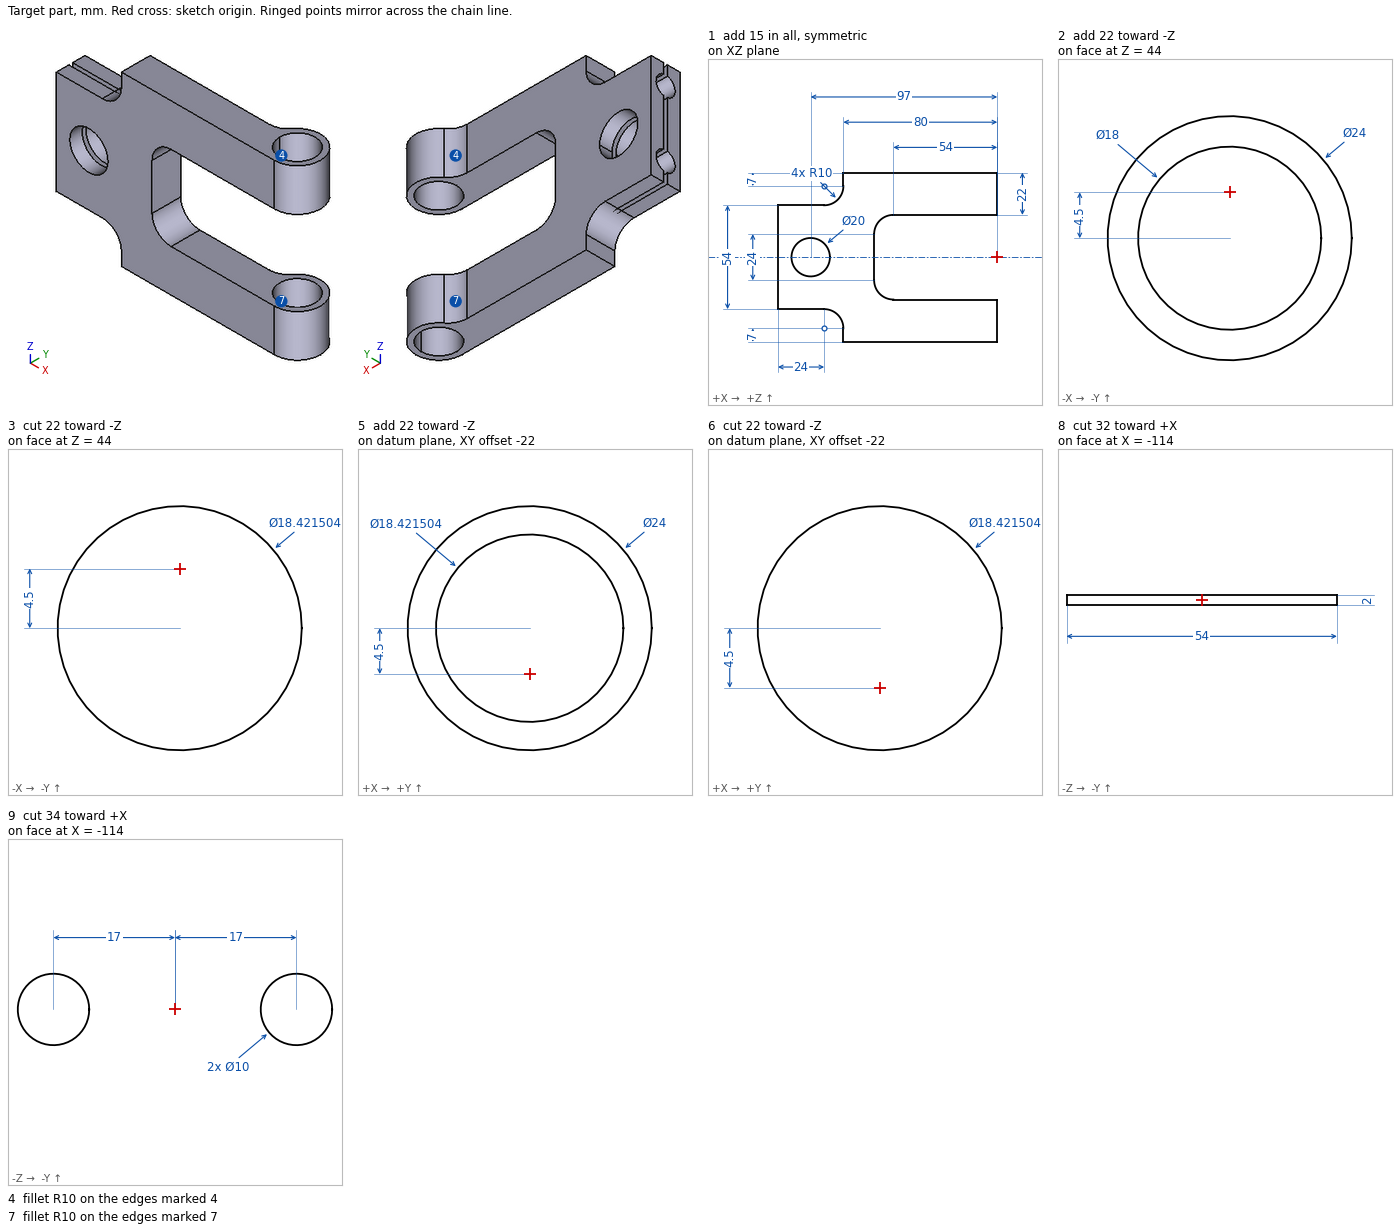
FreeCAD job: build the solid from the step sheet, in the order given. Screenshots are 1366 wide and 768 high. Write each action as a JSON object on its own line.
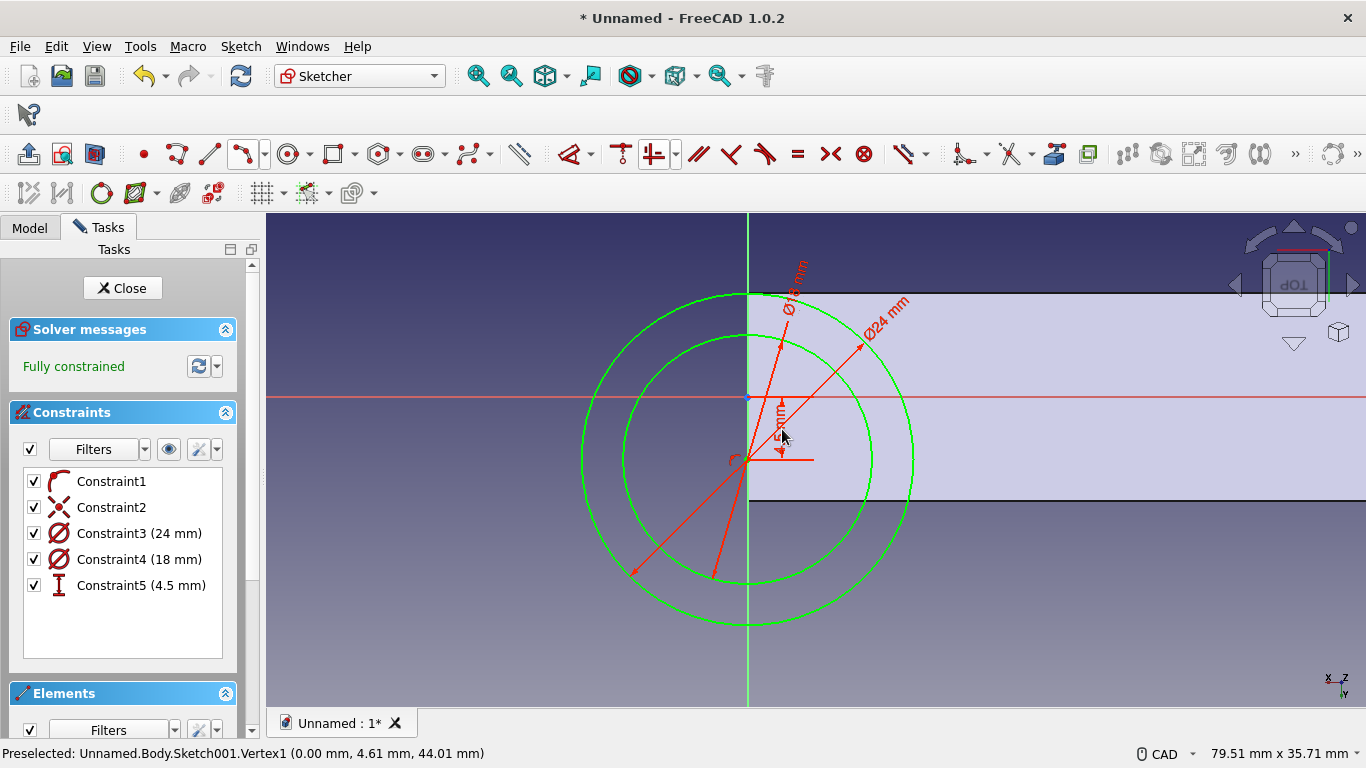
{"action": "left_click", "coordinate": [123, 288]}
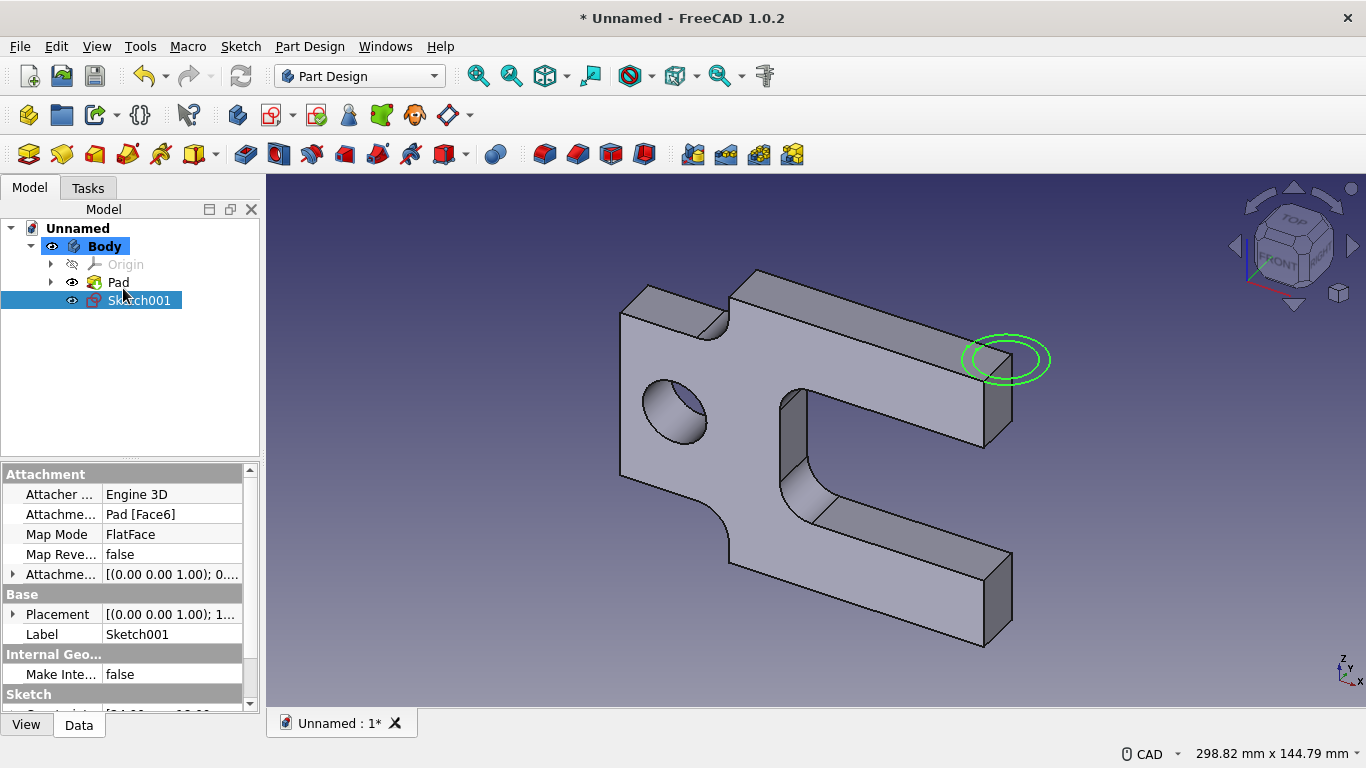
{"action": "left_click", "coordinate": [29, 154]}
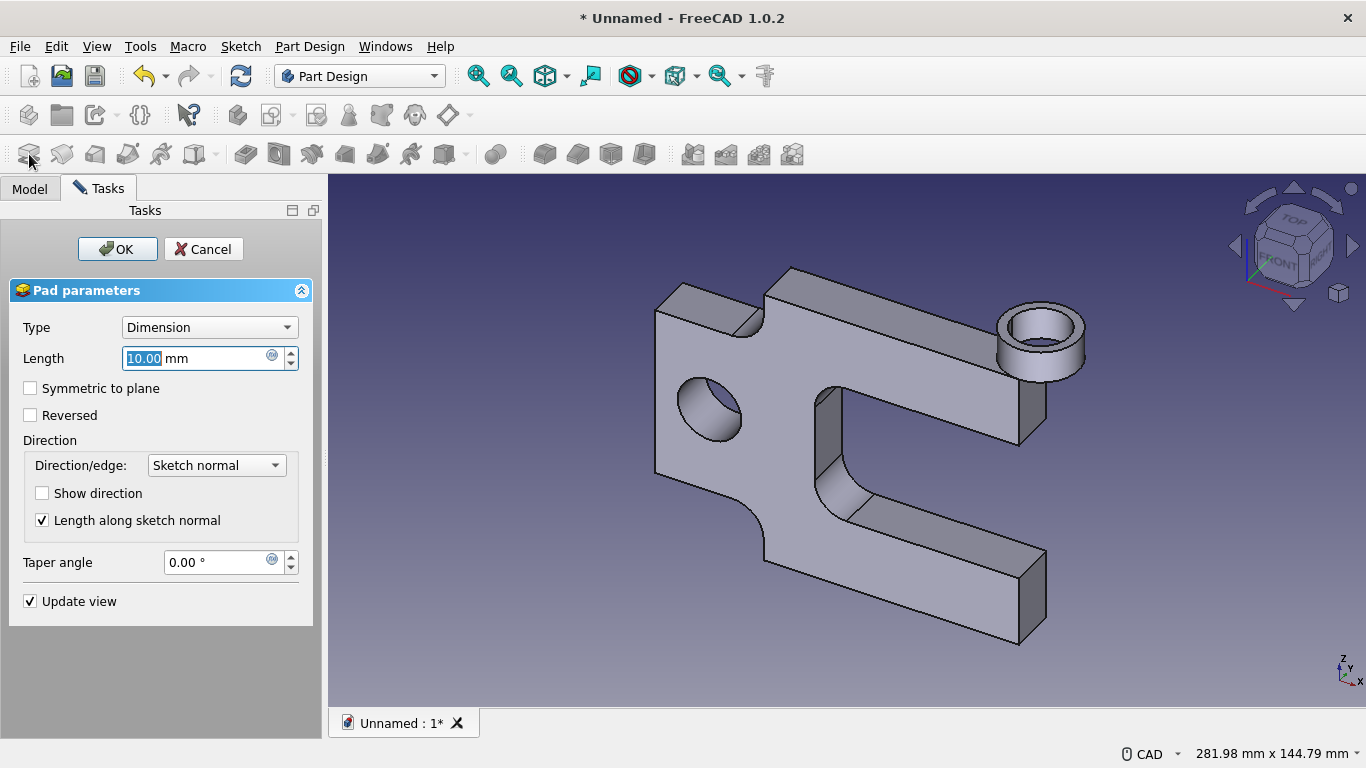
{"action": "type", "text": "22"}
{"action": "key", "text": "Tab"}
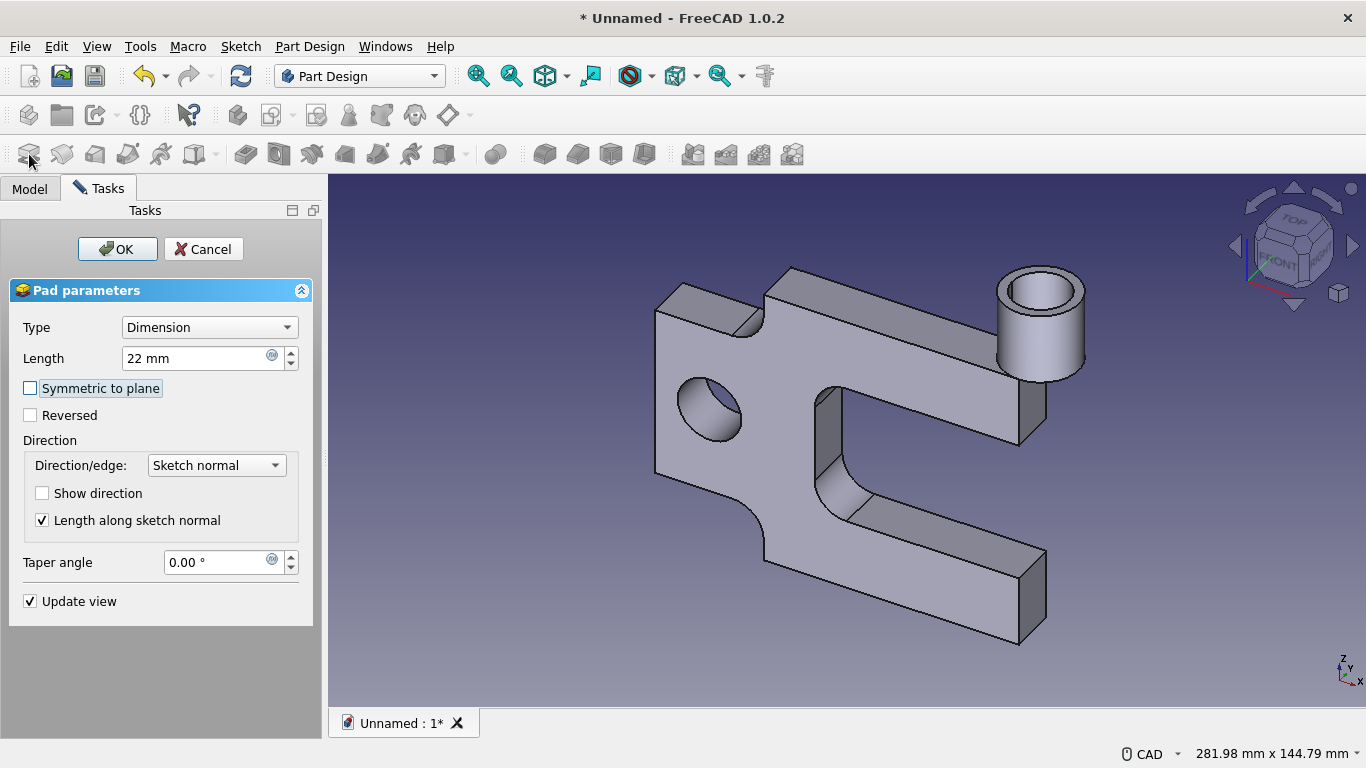
{"action": "left_click", "coordinate": [31, 415]}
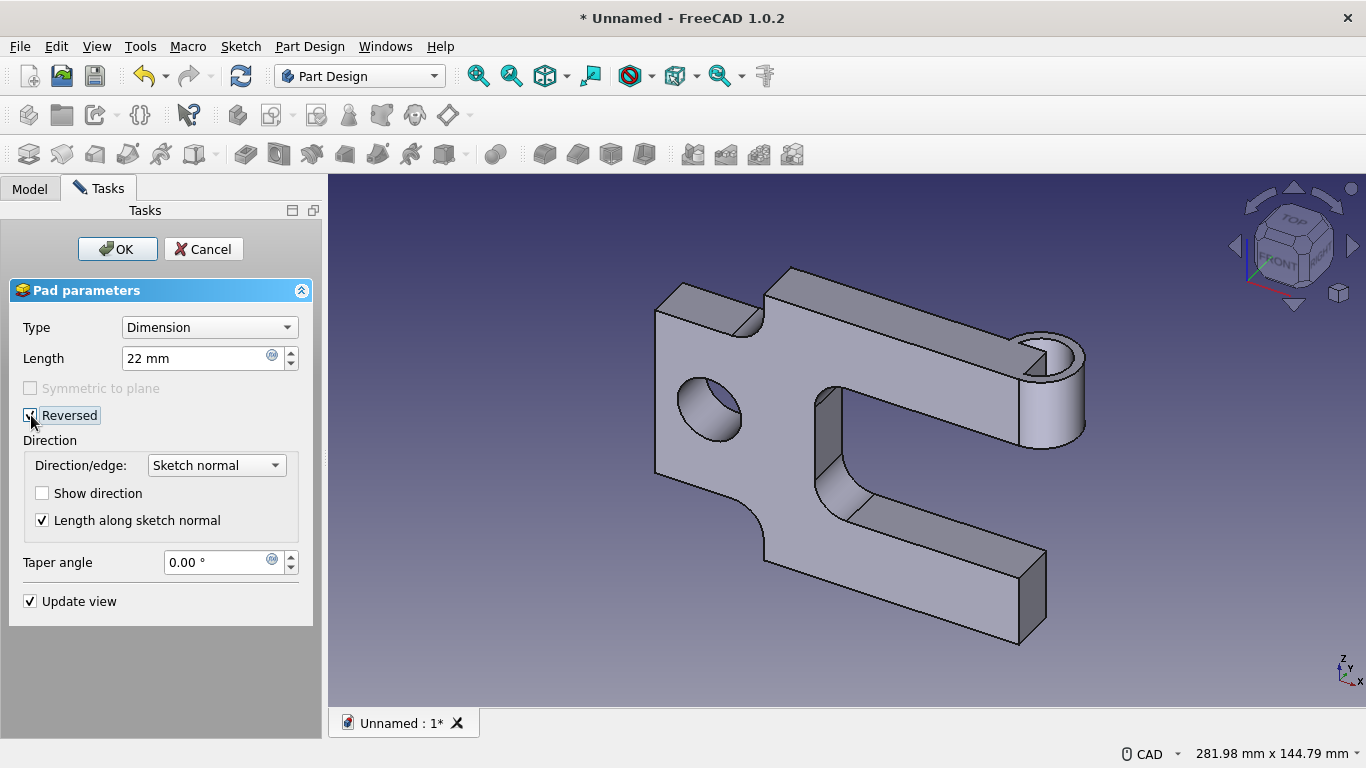
{"action": "left_click", "coordinate": [118, 249]}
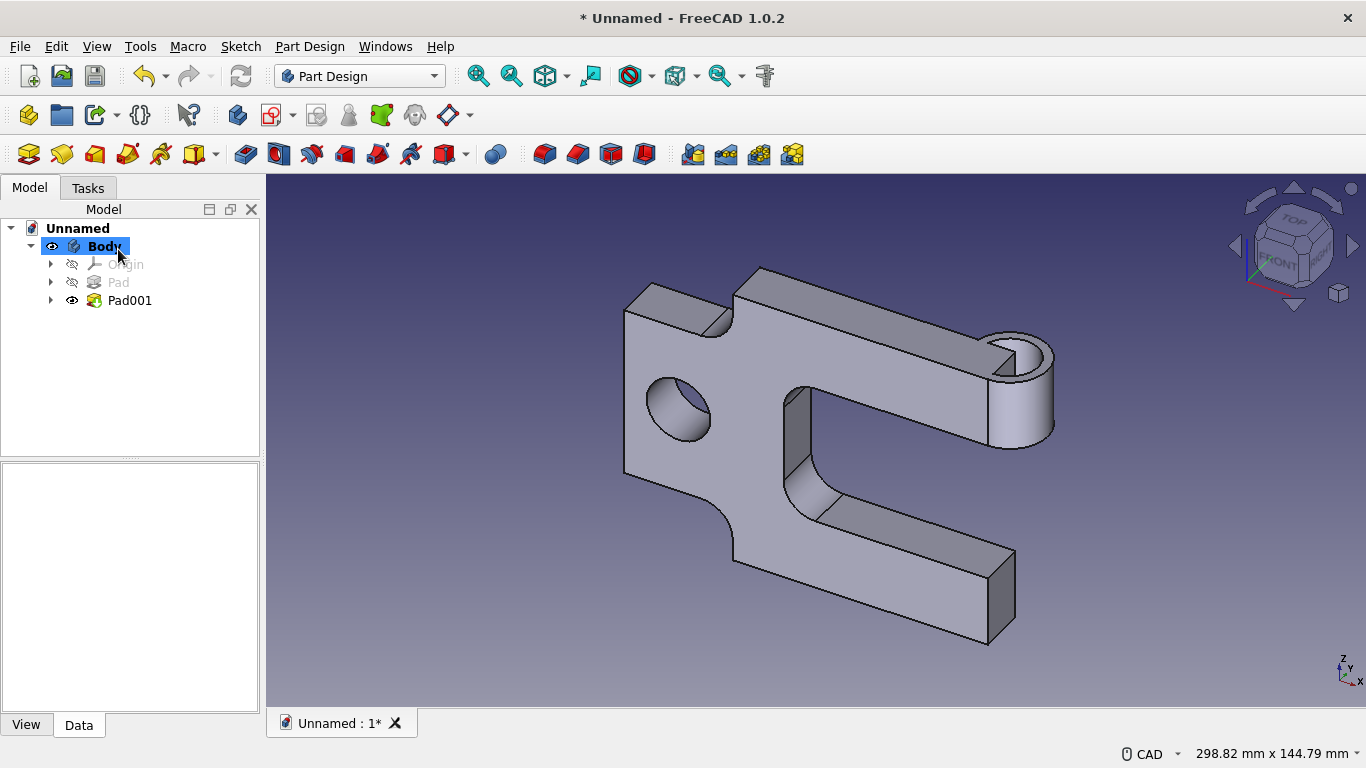
{"action": "left_click", "coordinate": [979, 355]}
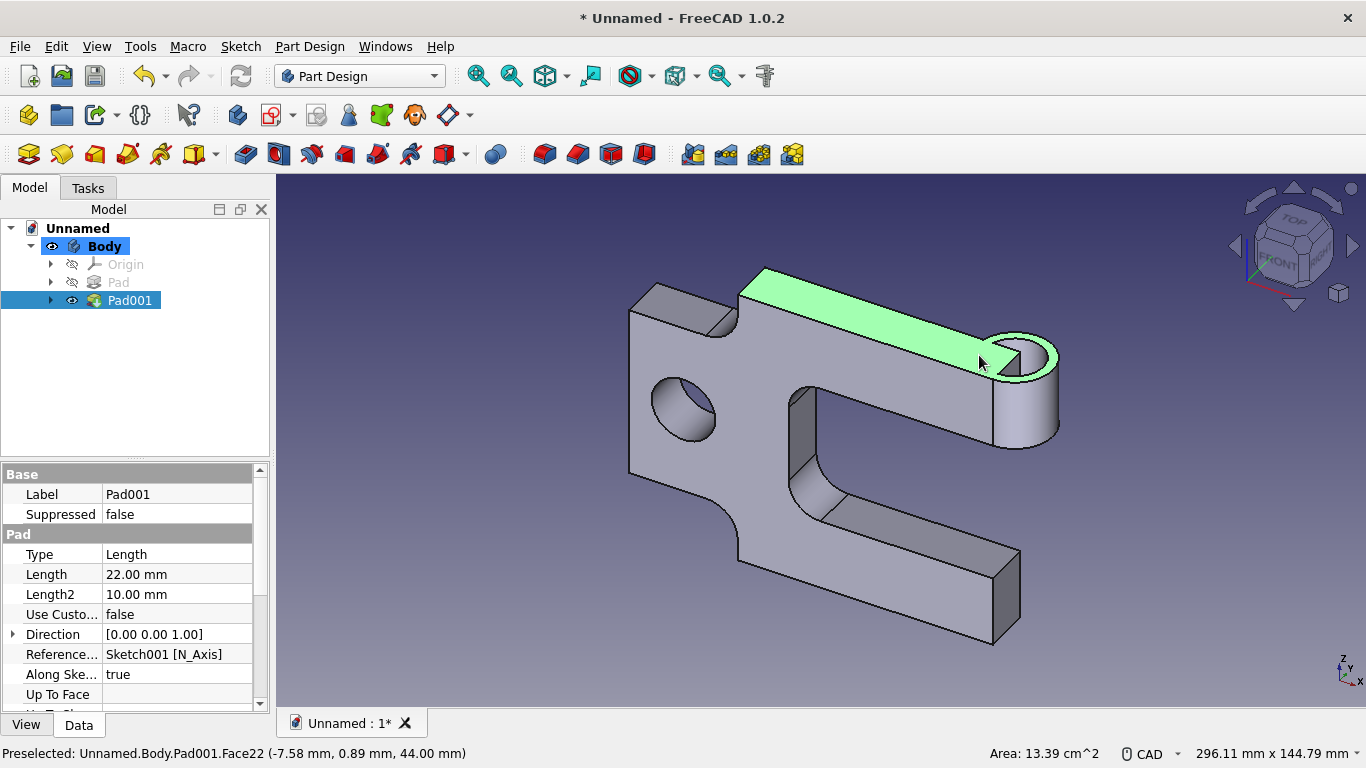
{"action": "left_click", "coordinate": [270, 116]}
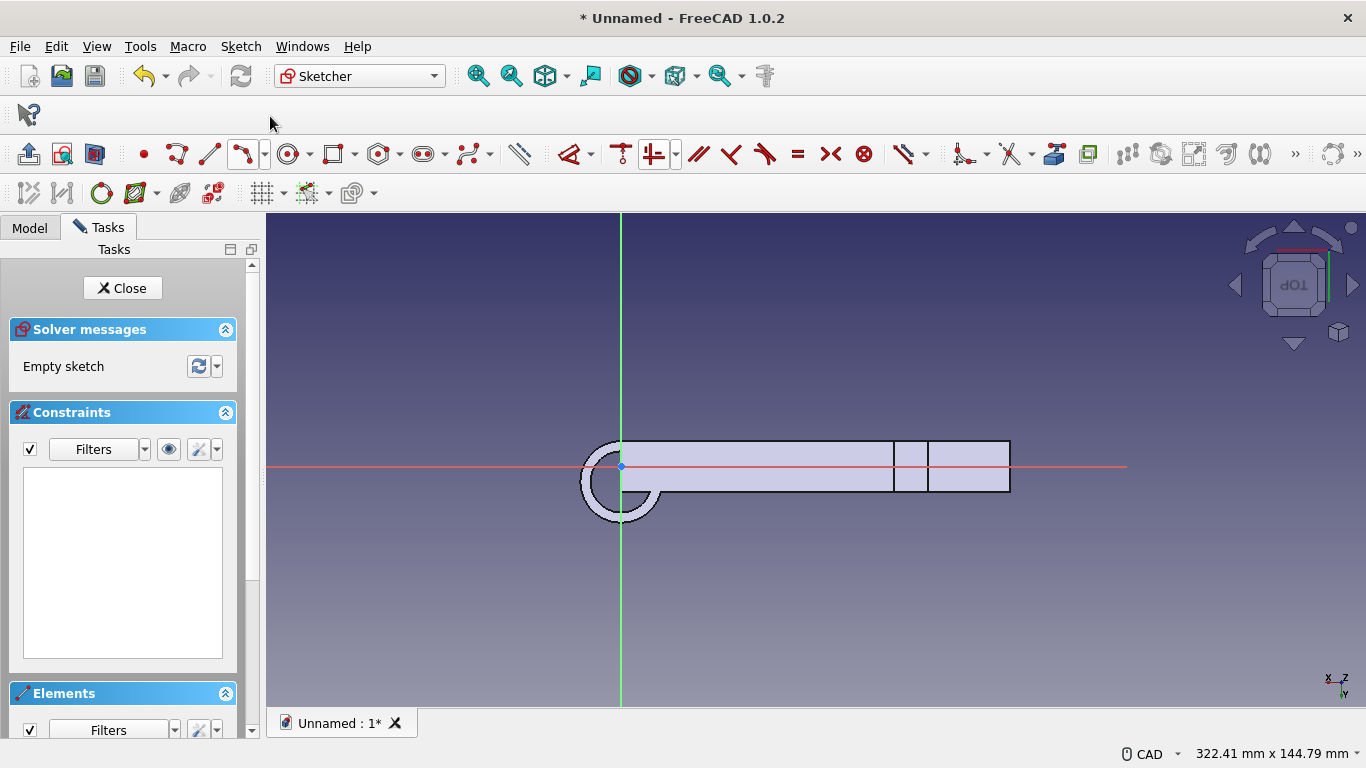
{"action": "scroll", "coordinate": [589, 487], "scroll_direction": "up", "scroll_amount": 8}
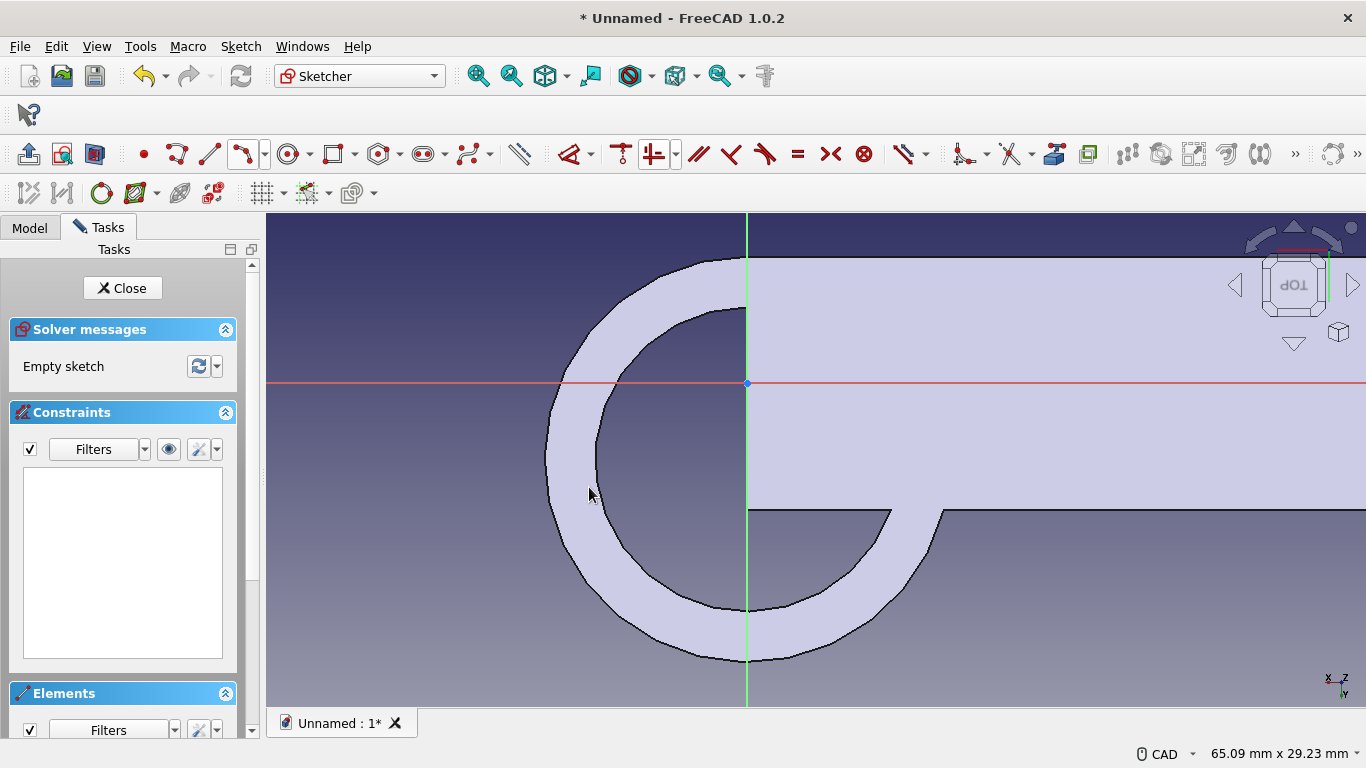
{"action": "left_click", "coordinate": [288, 154]}